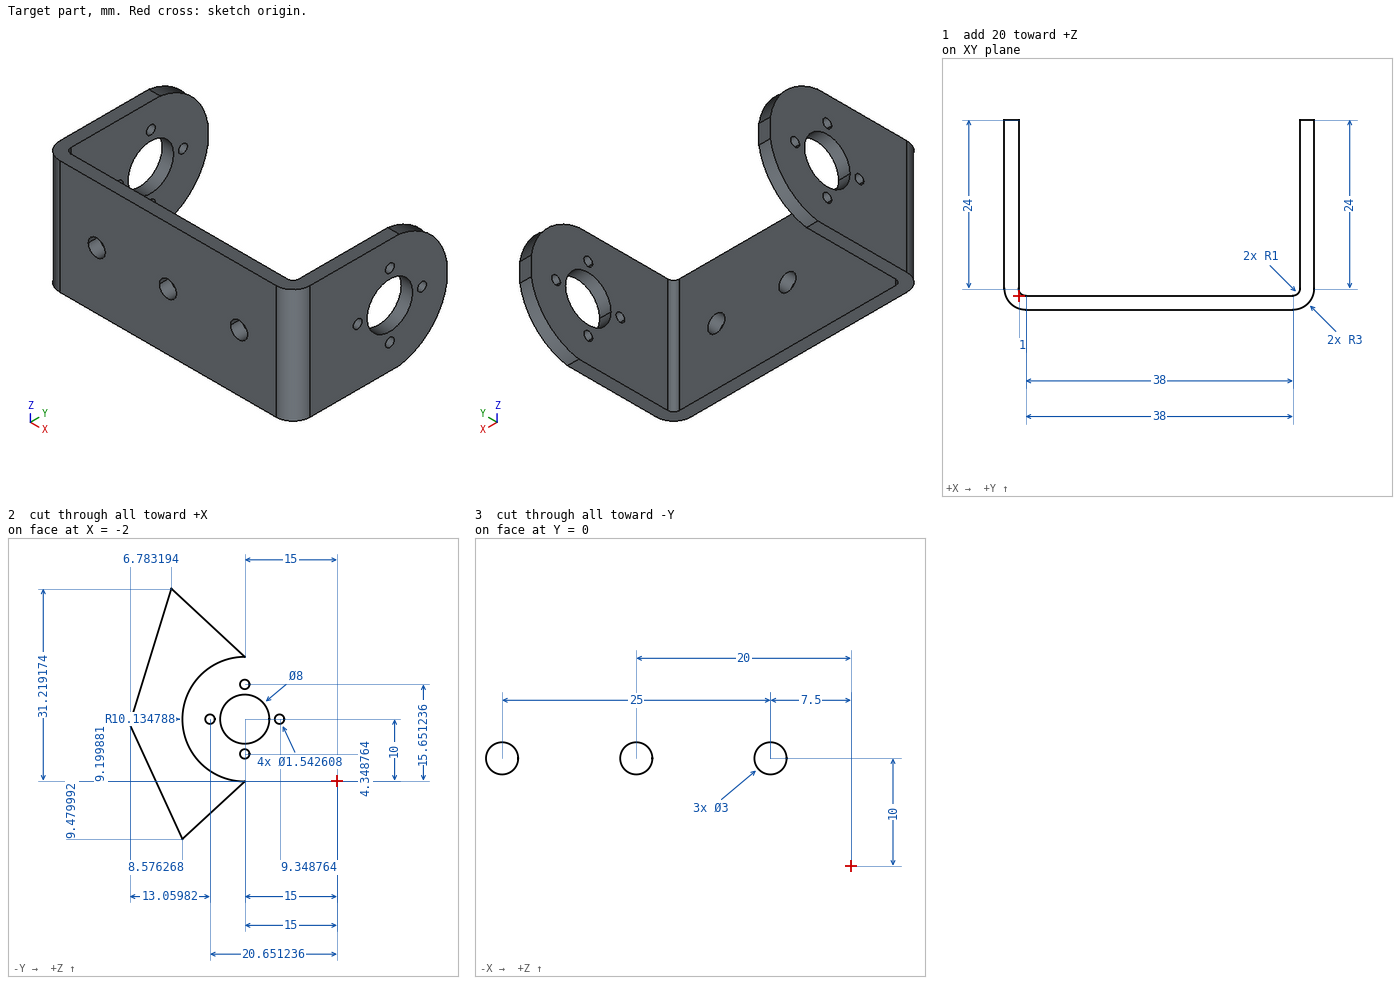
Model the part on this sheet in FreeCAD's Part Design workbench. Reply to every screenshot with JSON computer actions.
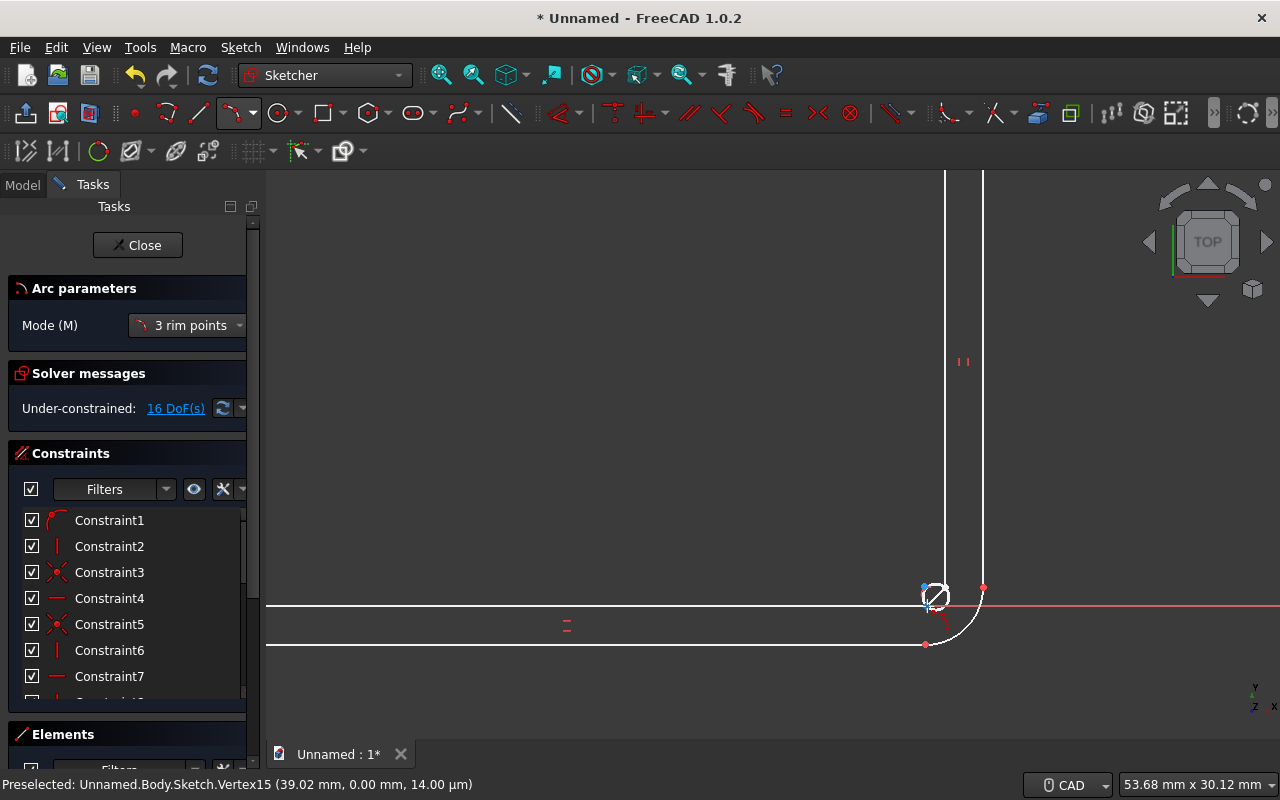
{"action": "scroll", "coordinate": [940, 601], "scroll_direction": "up", "scroll_amount": 6}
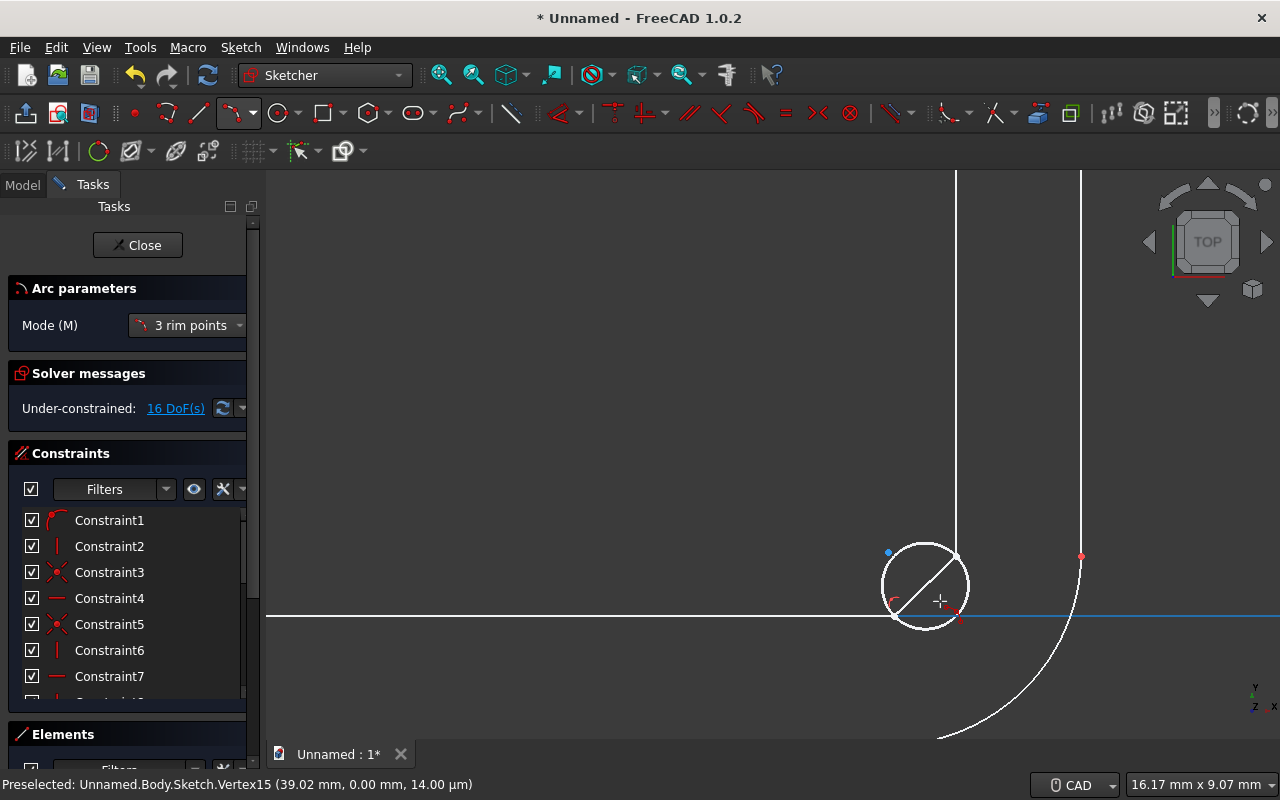
{"action": "left_click", "coordinate": [938, 598]}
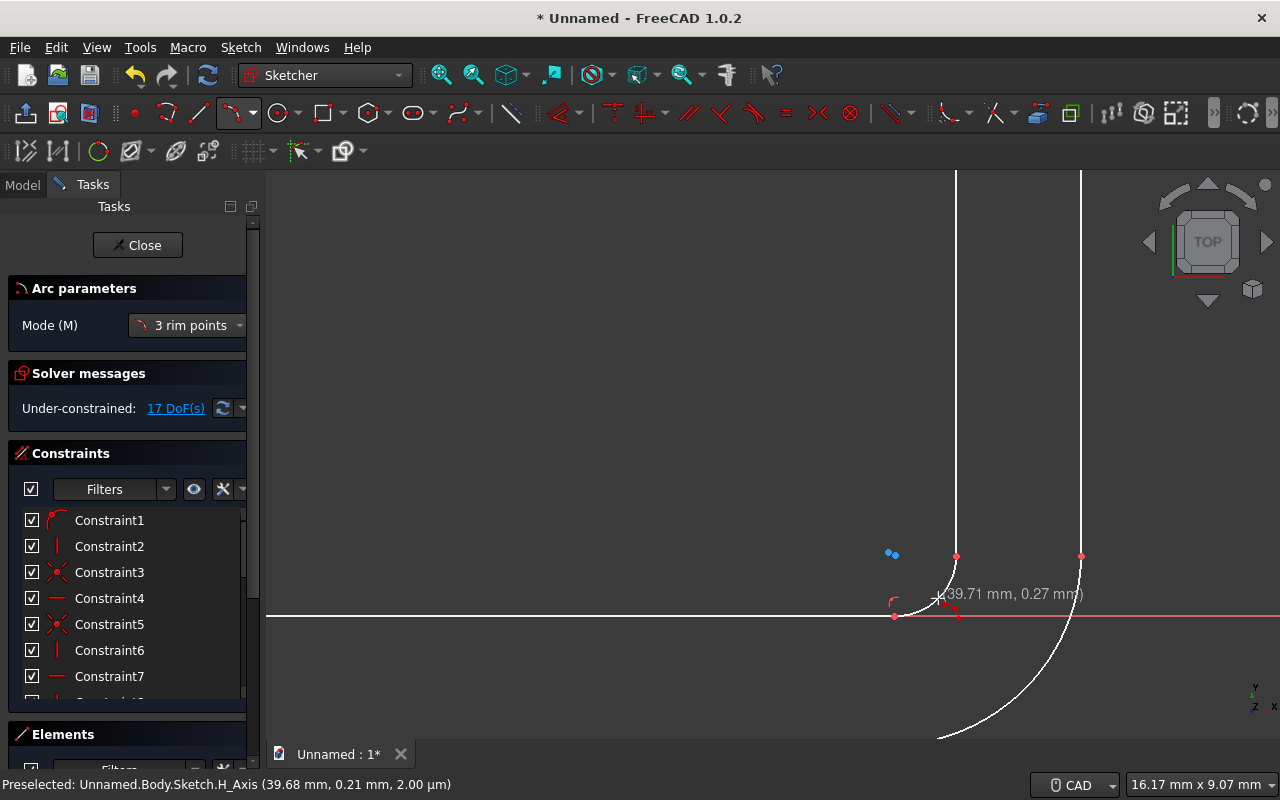
{"action": "scroll", "coordinate": [958, 596], "scroll_direction": "down", "scroll_amount": 8}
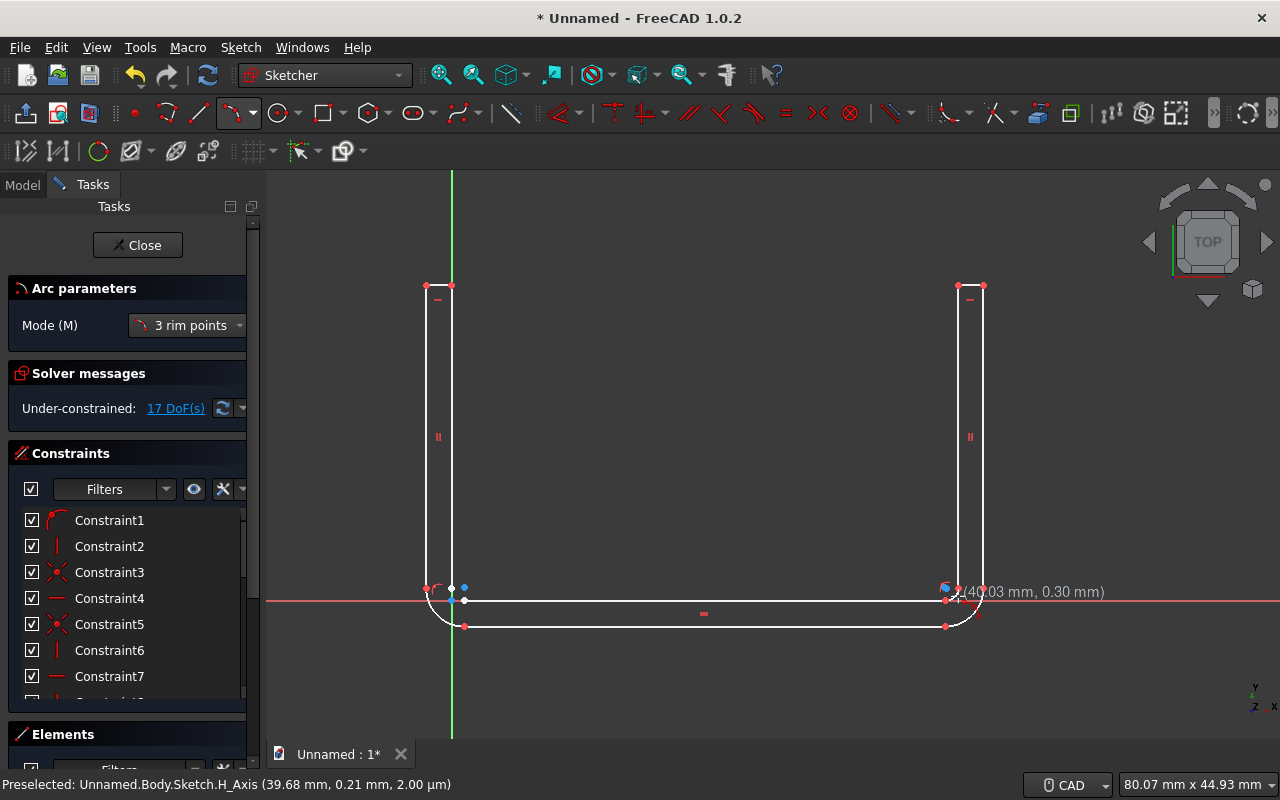
{"action": "scroll", "coordinate": [464, 601], "scroll_direction": "up", "scroll_amount": 2}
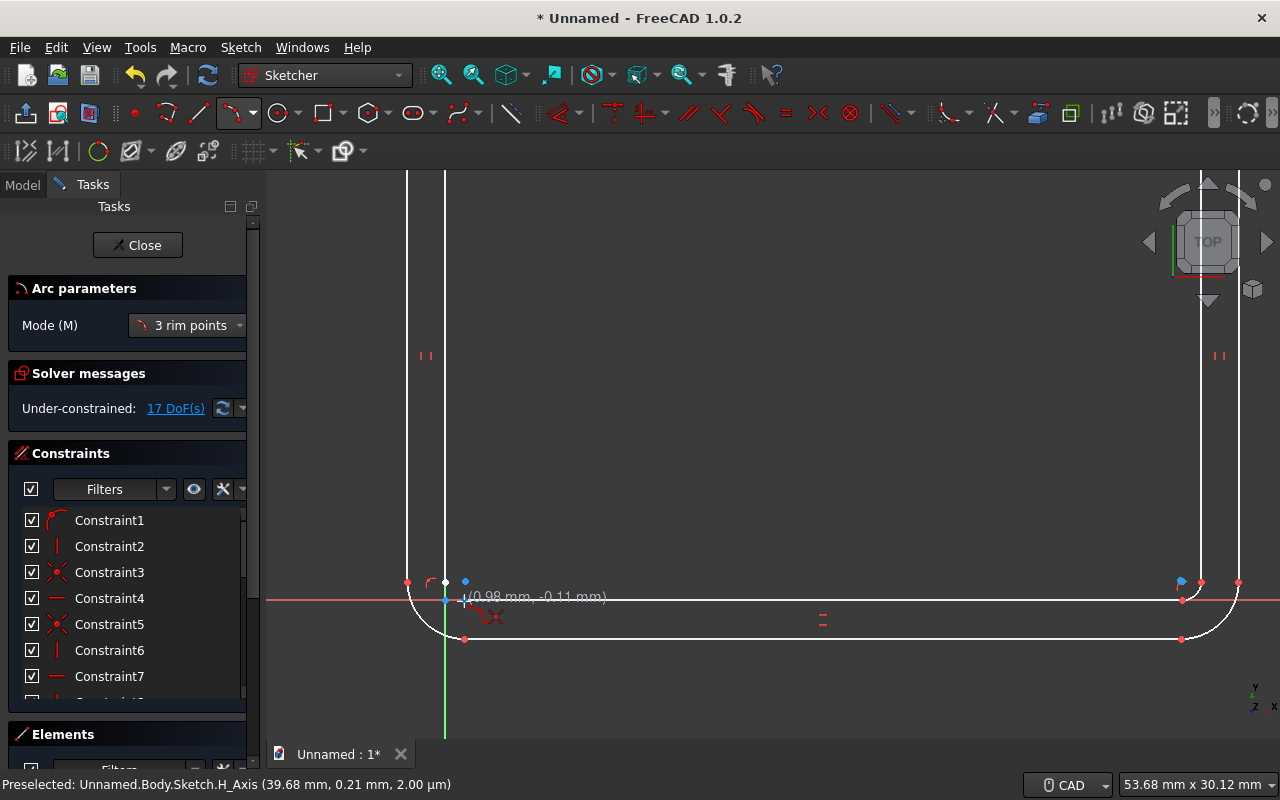
{"action": "left_click", "coordinate": [464, 591]}
{"action": "left_click", "coordinate": [445, 582]}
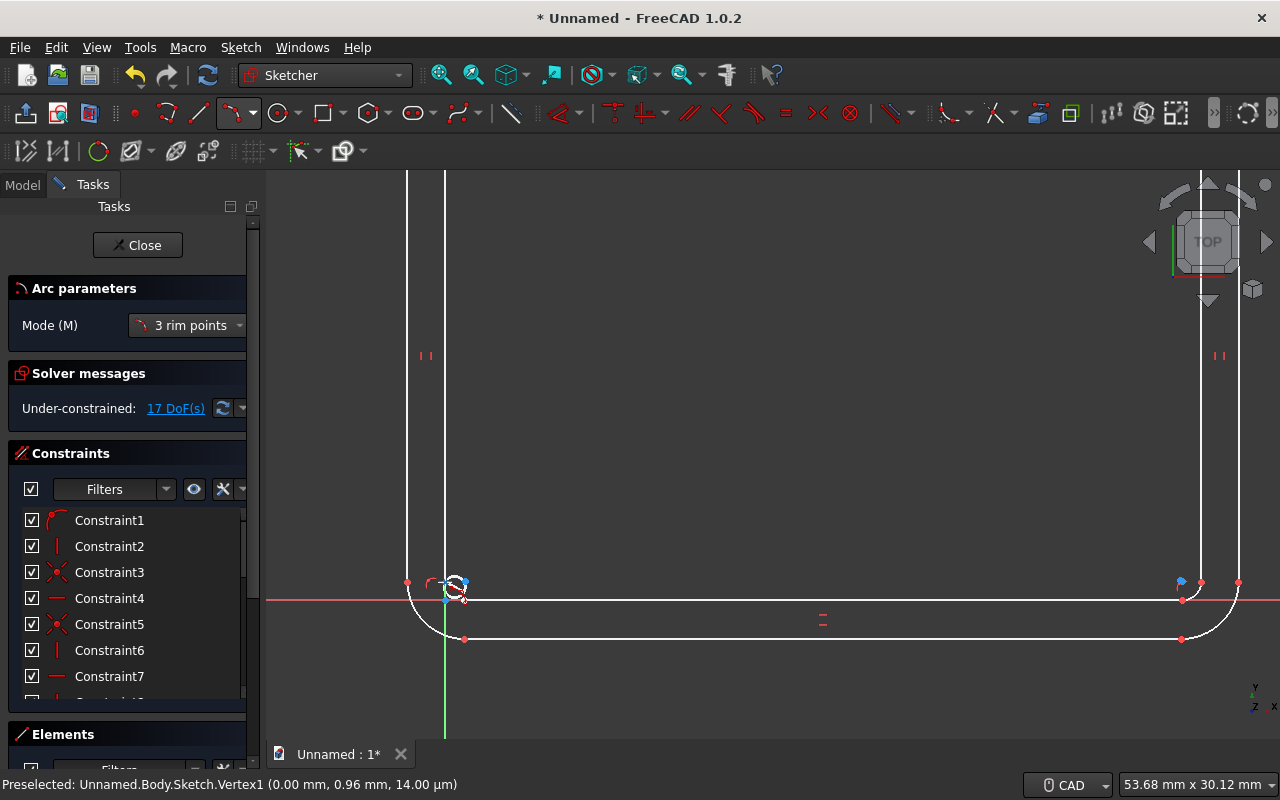
{"action": "scroll", "coordinate": [451, 595], "scroll_direction": "up", "scroll_amount": 6}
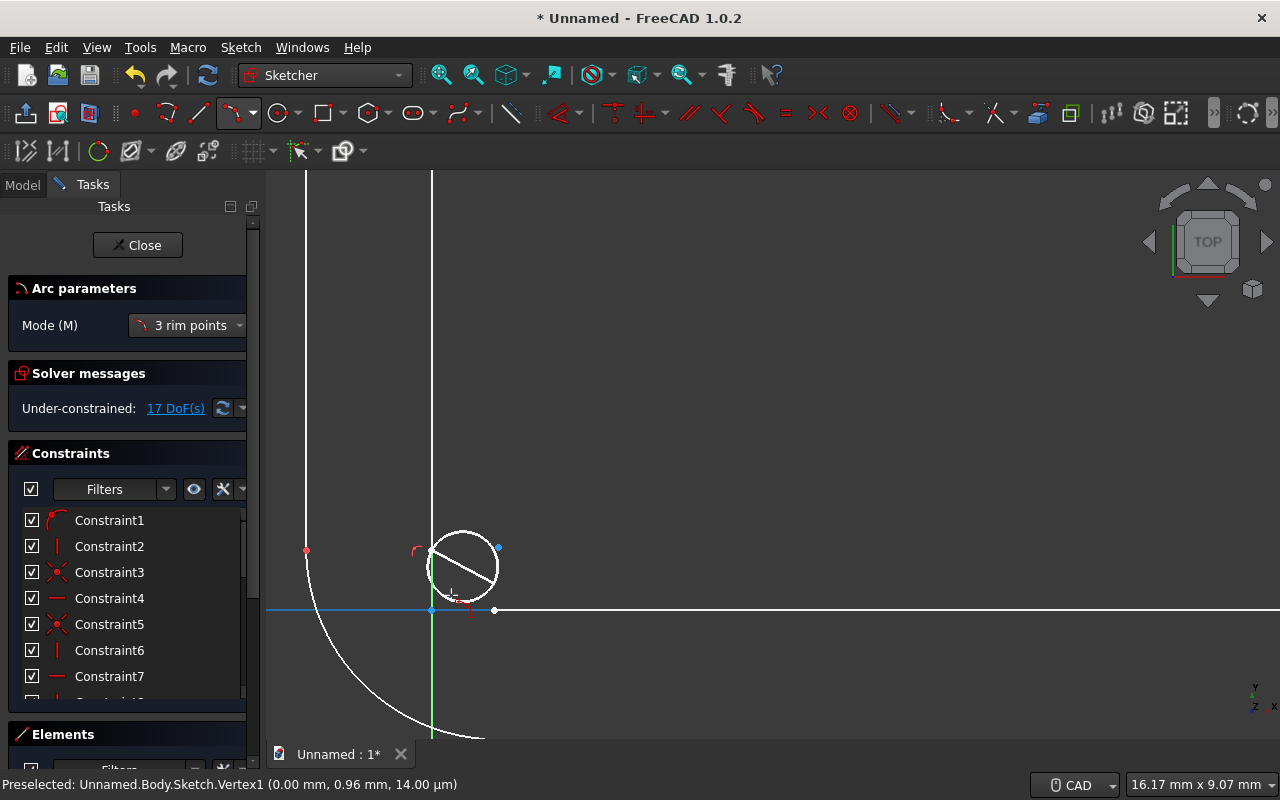
{"action": "left_click", "coordinate": [450, 592]}
{"action": "key", "text": "Escape"}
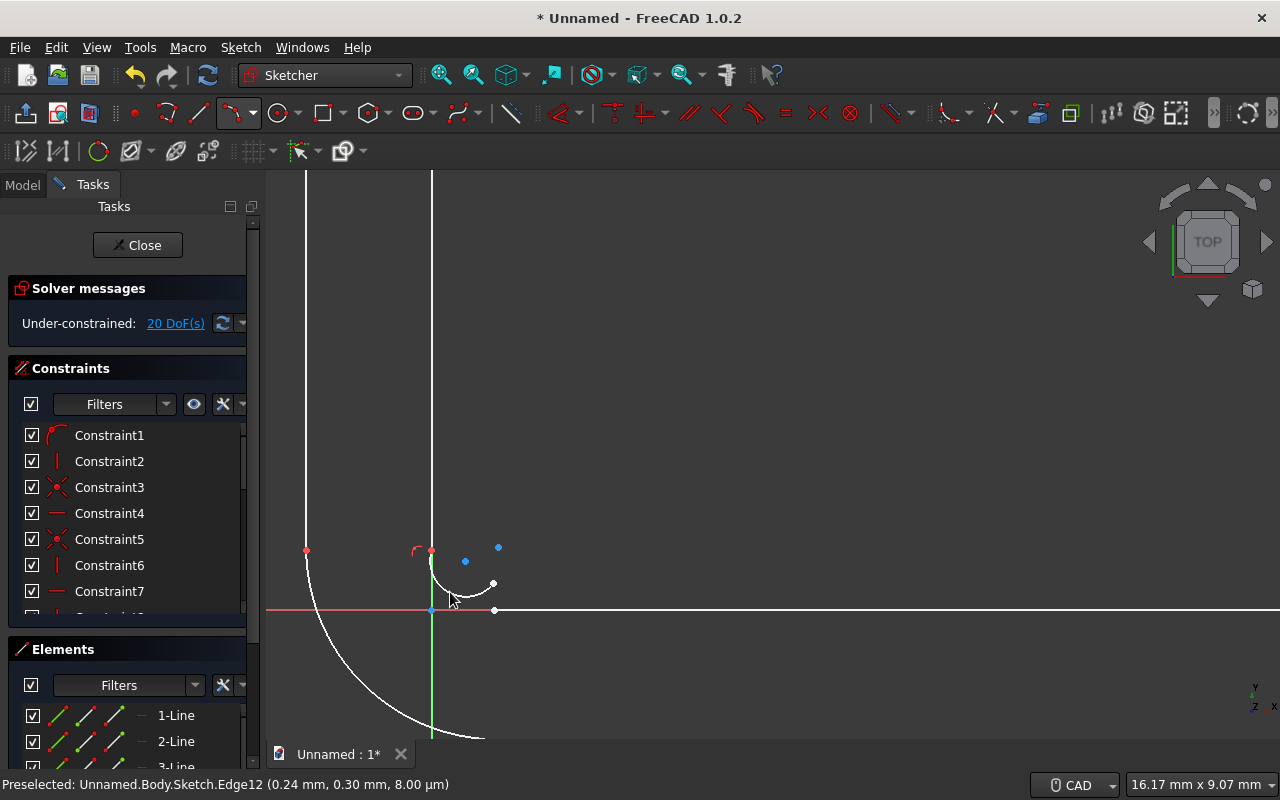
{"action": "scroll", "coordinate": [456, 598], "scroll_direction": "down", "scroll_amount": 8}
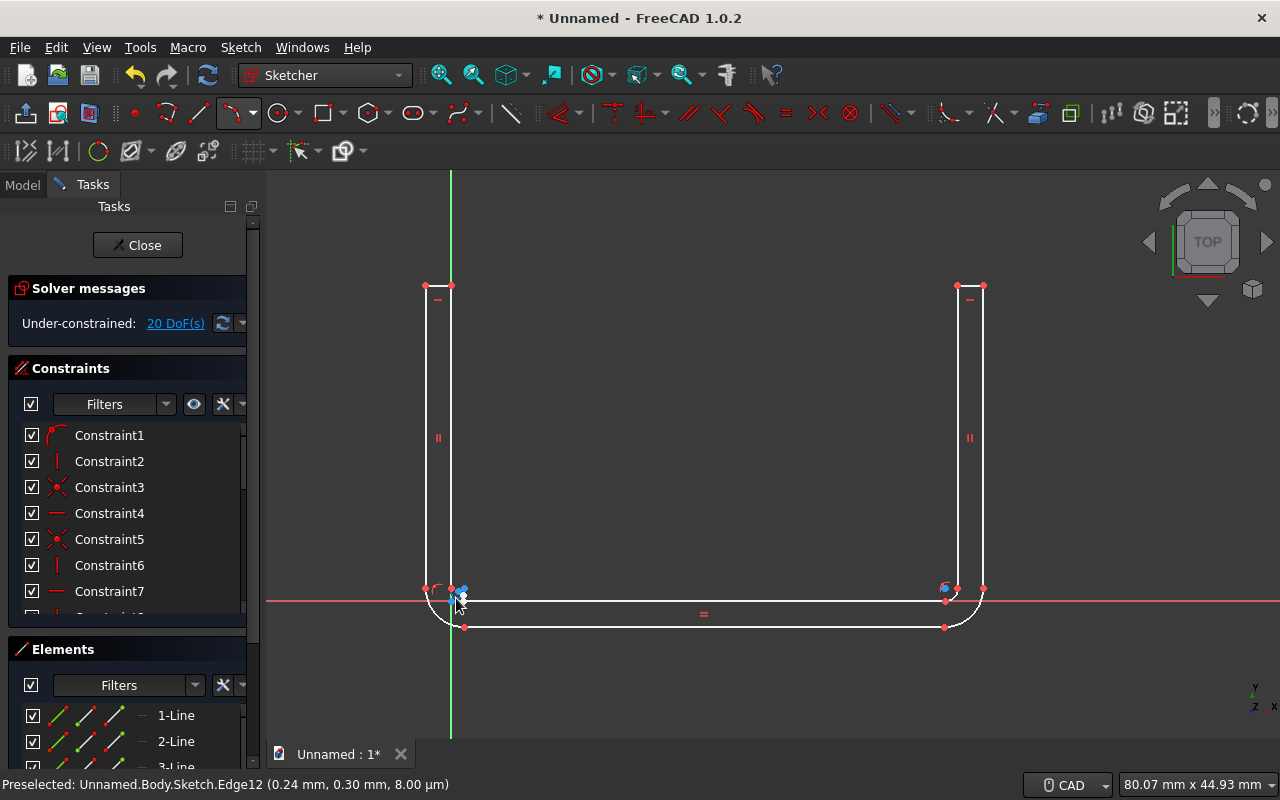
{"action": "left_click", "coordinate": [451, 528]}